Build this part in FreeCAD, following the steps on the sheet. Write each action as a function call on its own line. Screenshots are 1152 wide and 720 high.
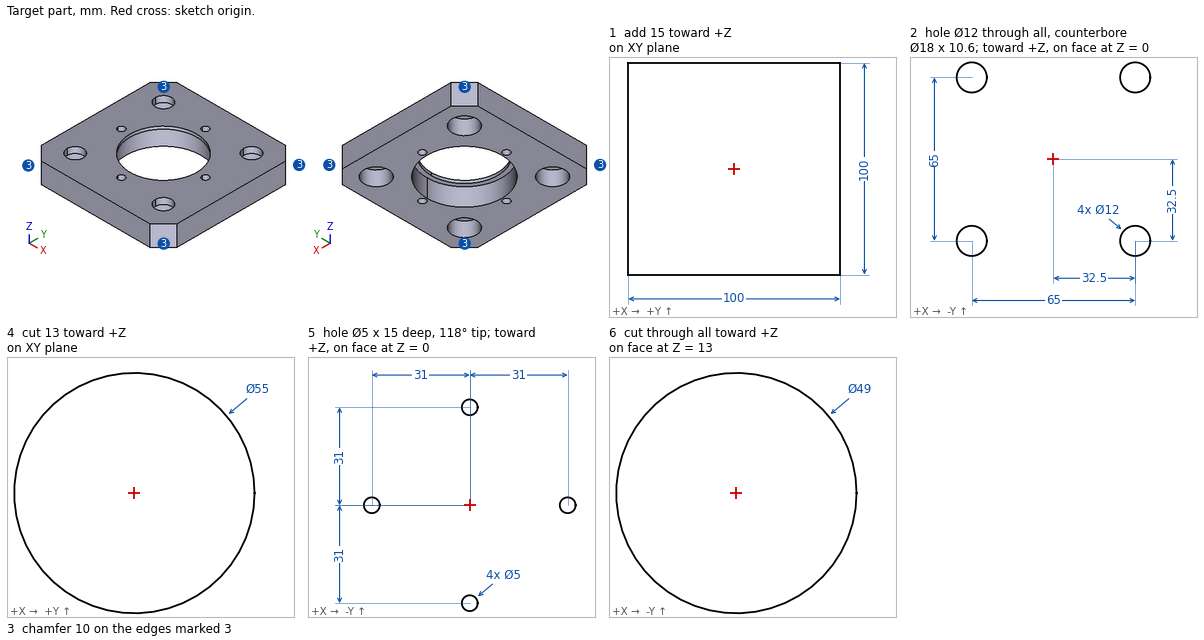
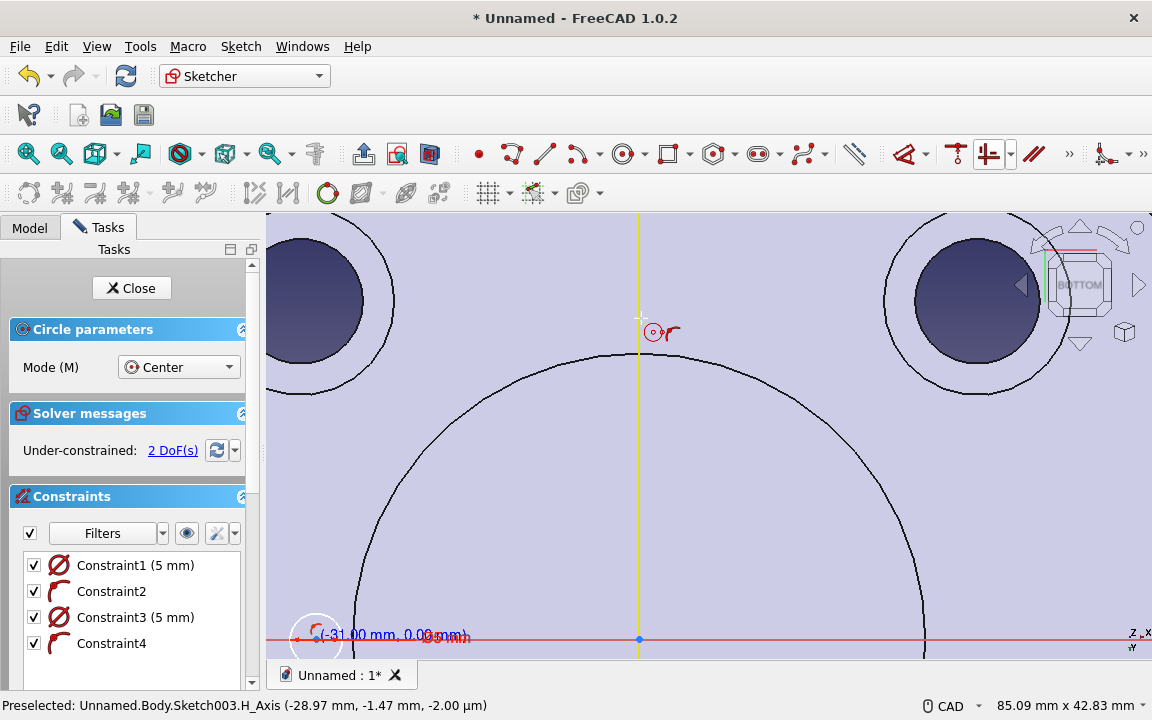
click(639, 317)
move(657, 299)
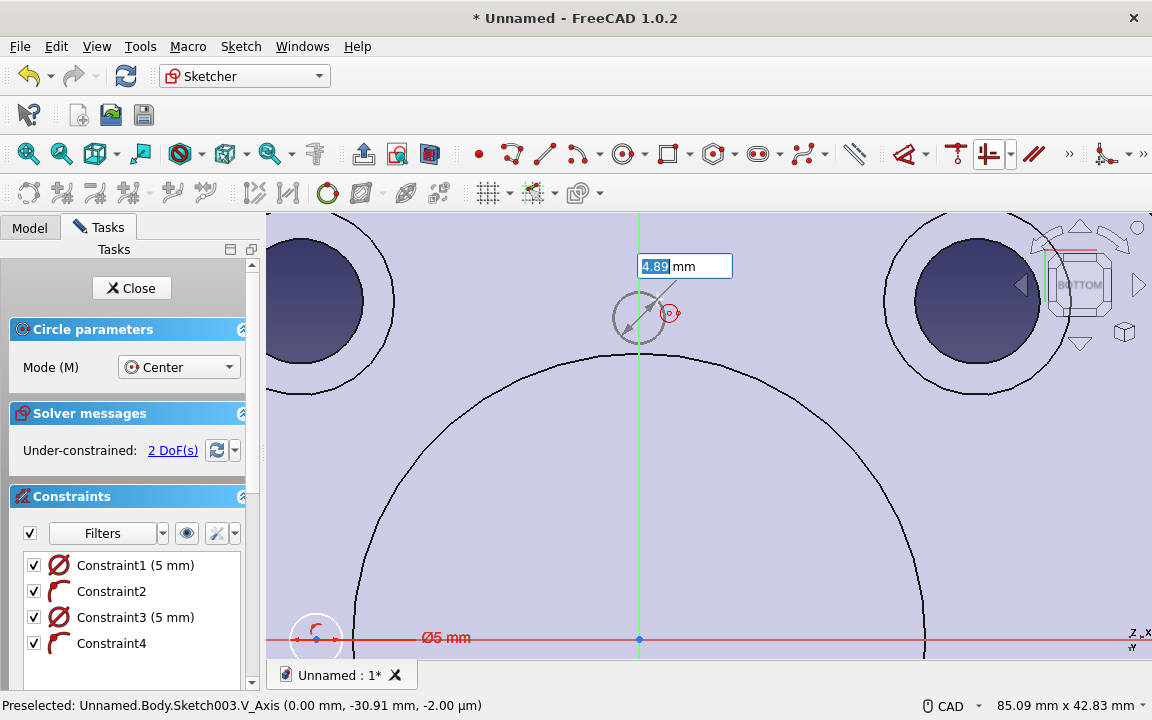
text(5)
key(Return)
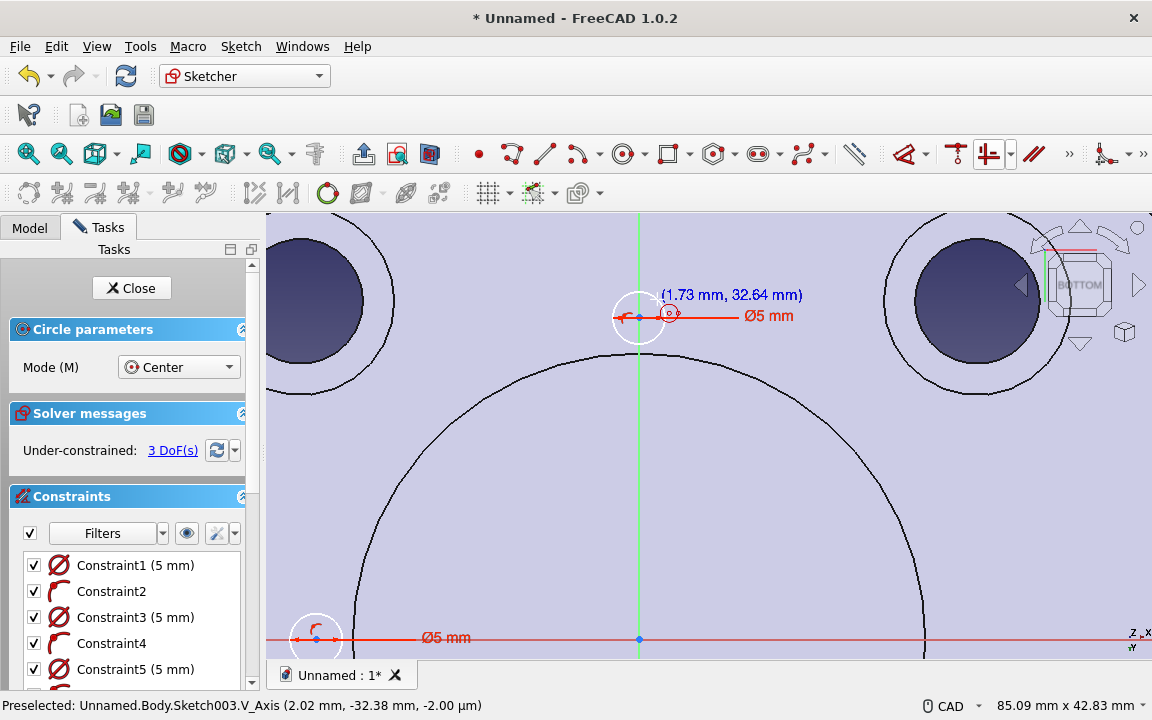
scroll(641, 317, down, 5)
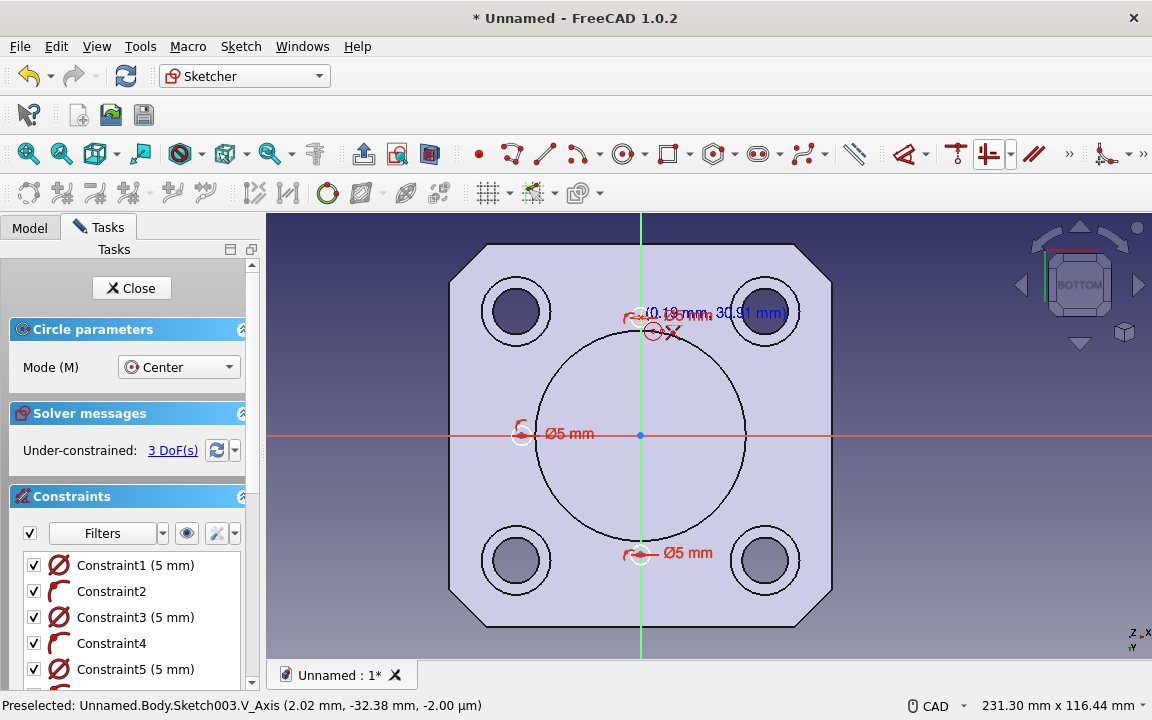
scroll(759, 436, up, 5)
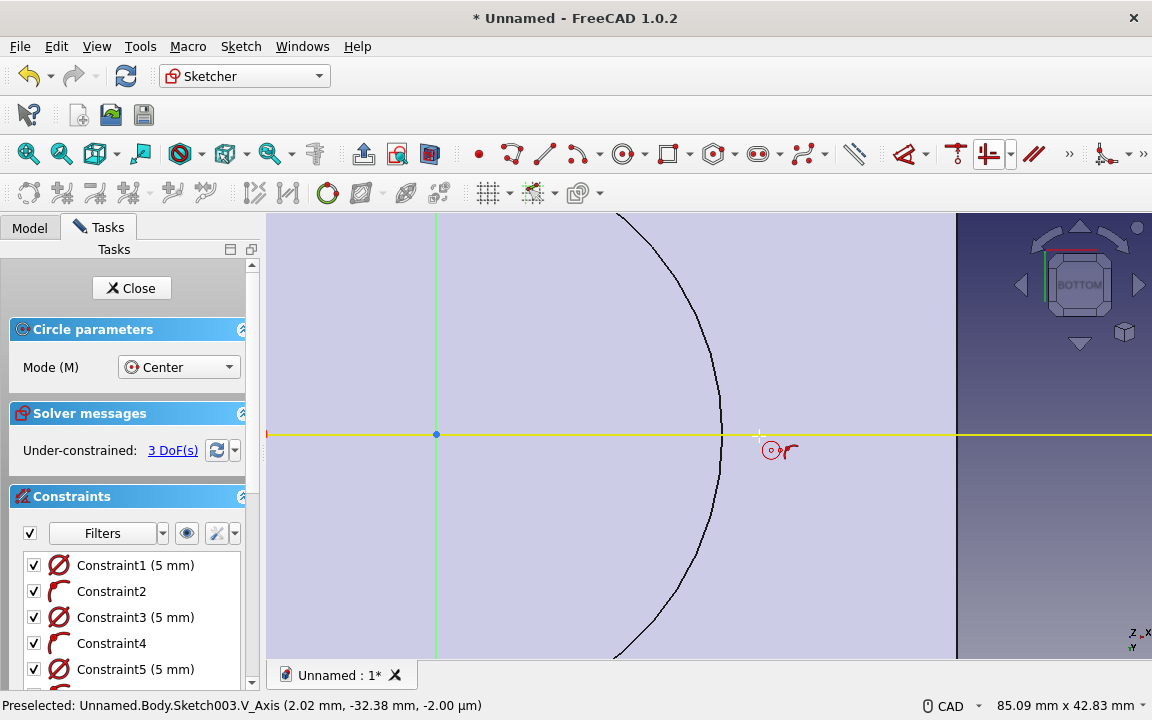
click(759, 435)
move(777, 416)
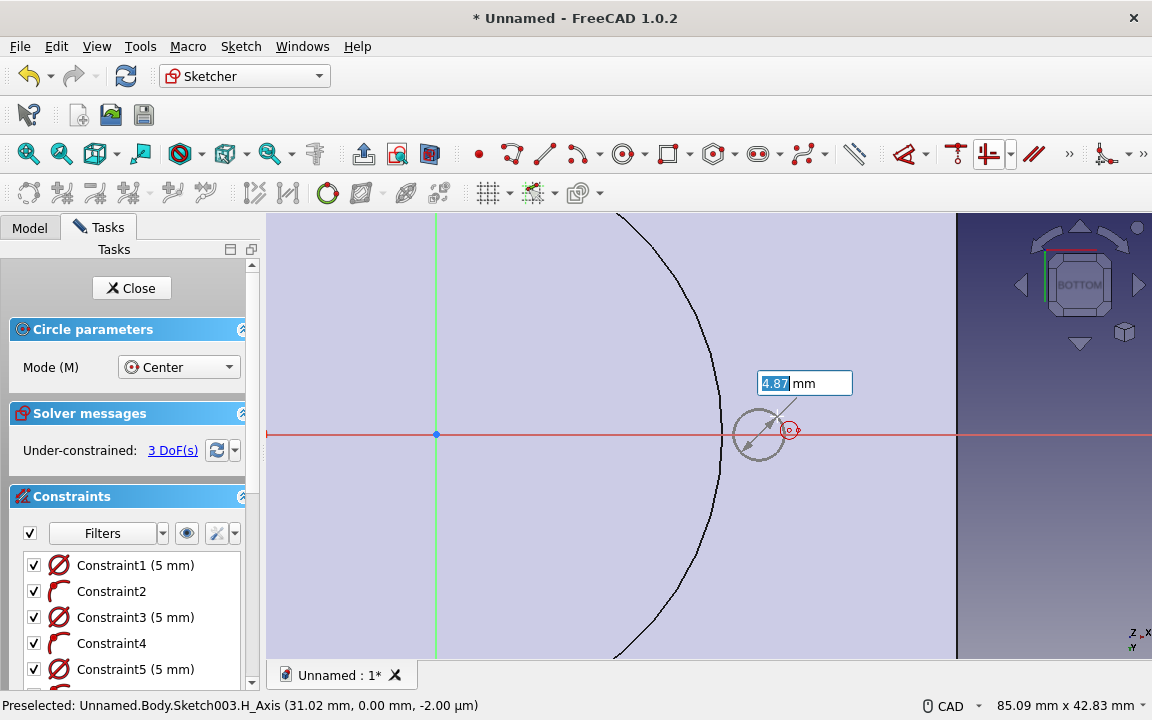
text(5)
key(Return)
key(Escape)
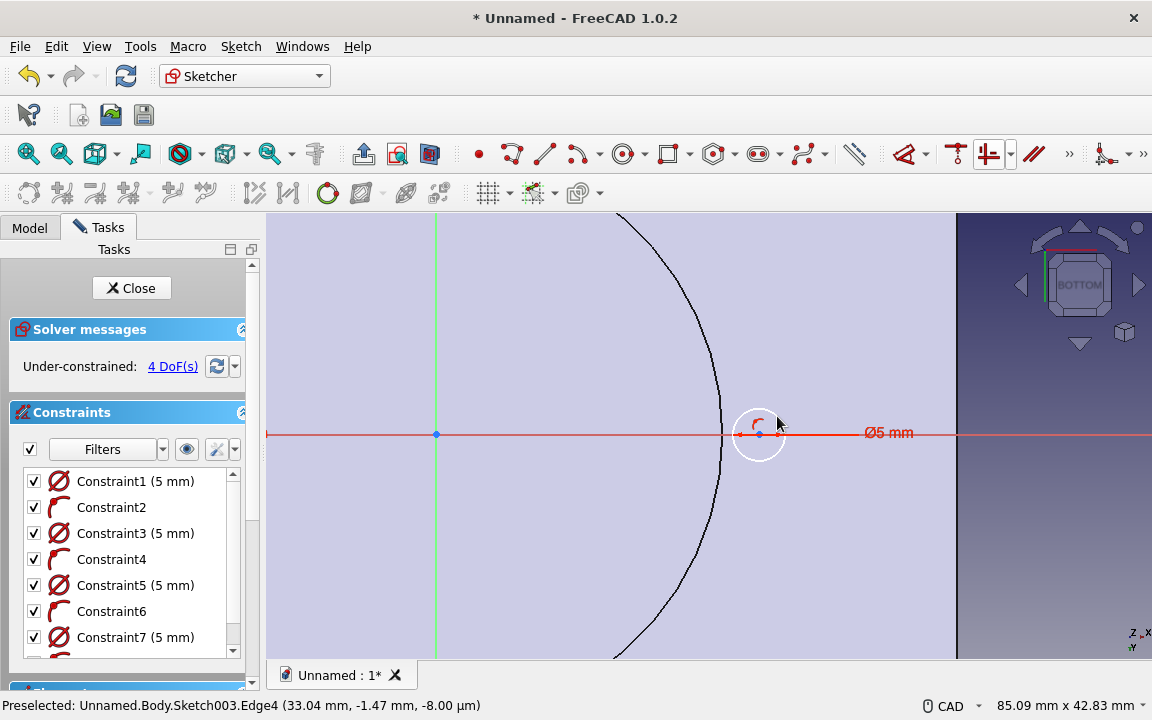
click(904, 154)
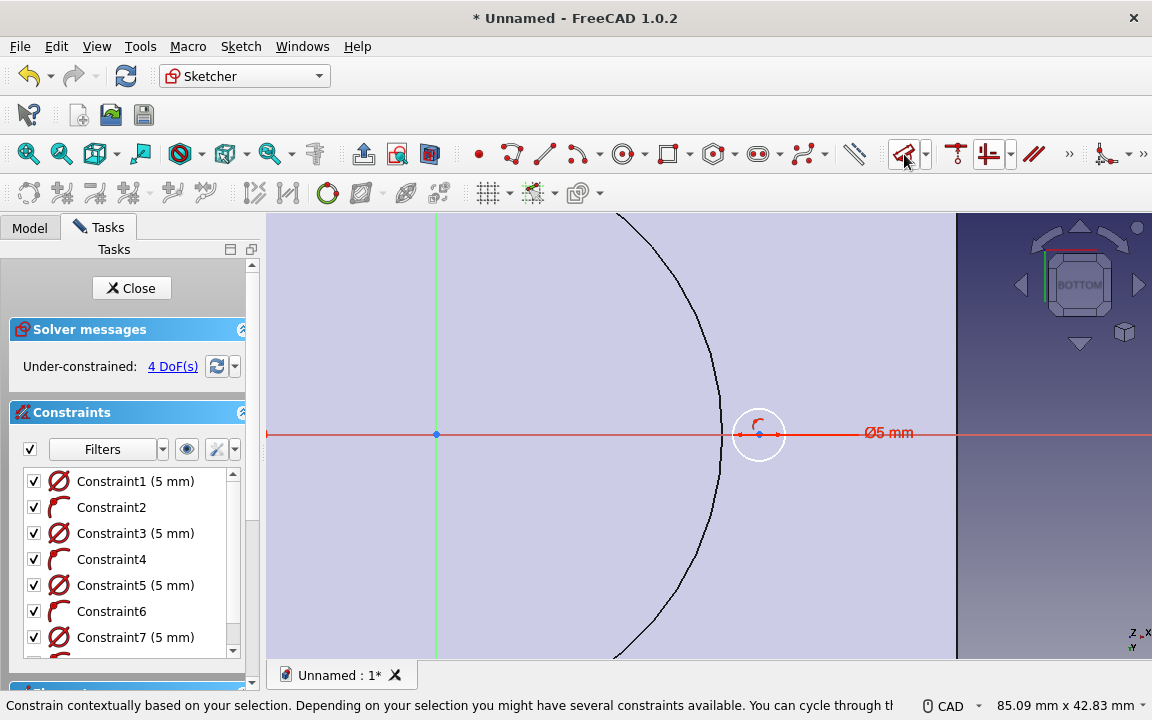
scroll(759, 437, down, 5)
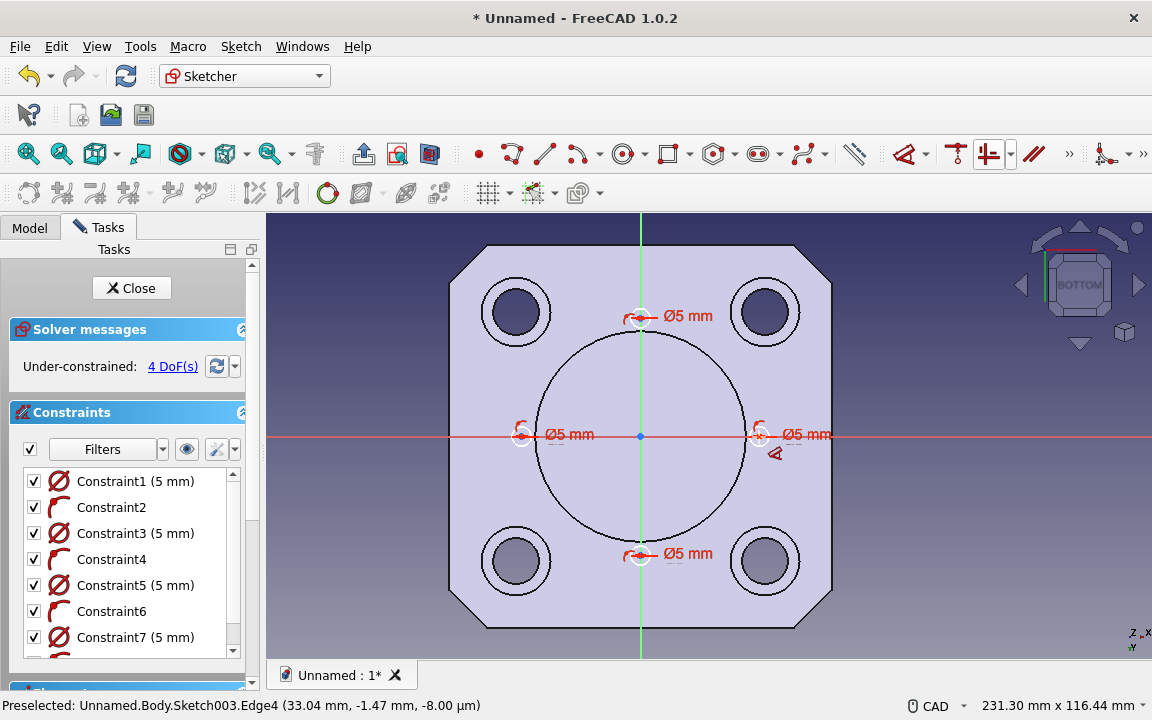
click(641, 556)
click(675, 496)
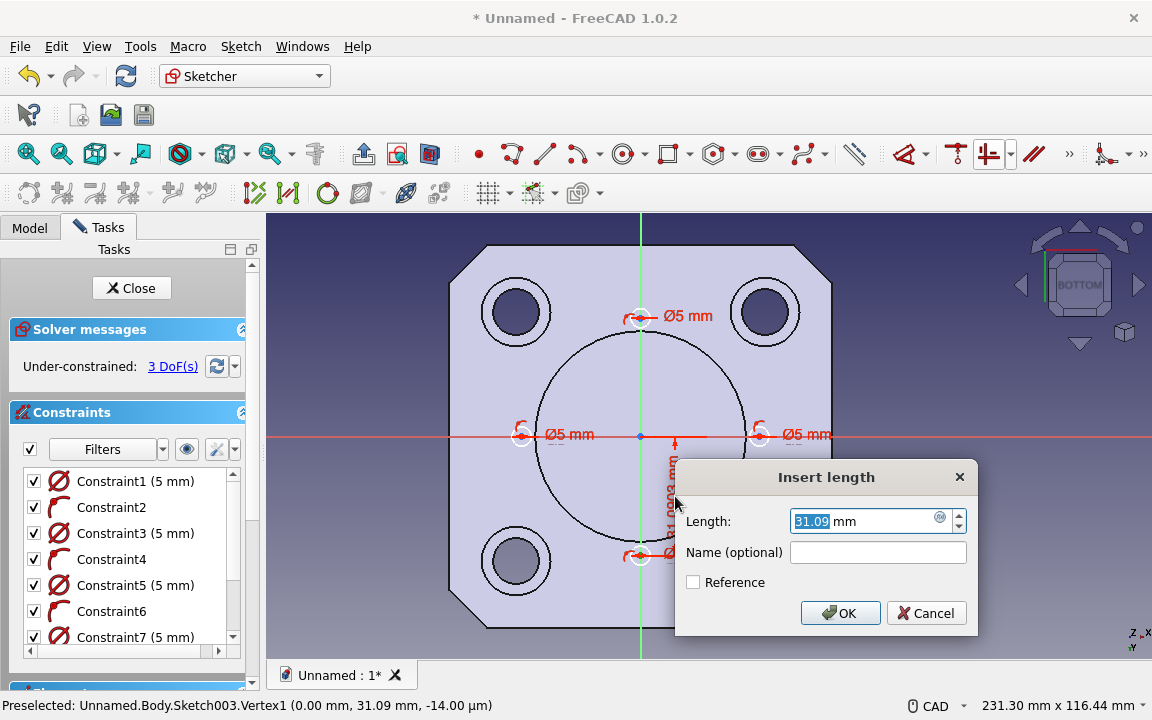
text(31)
key(Return)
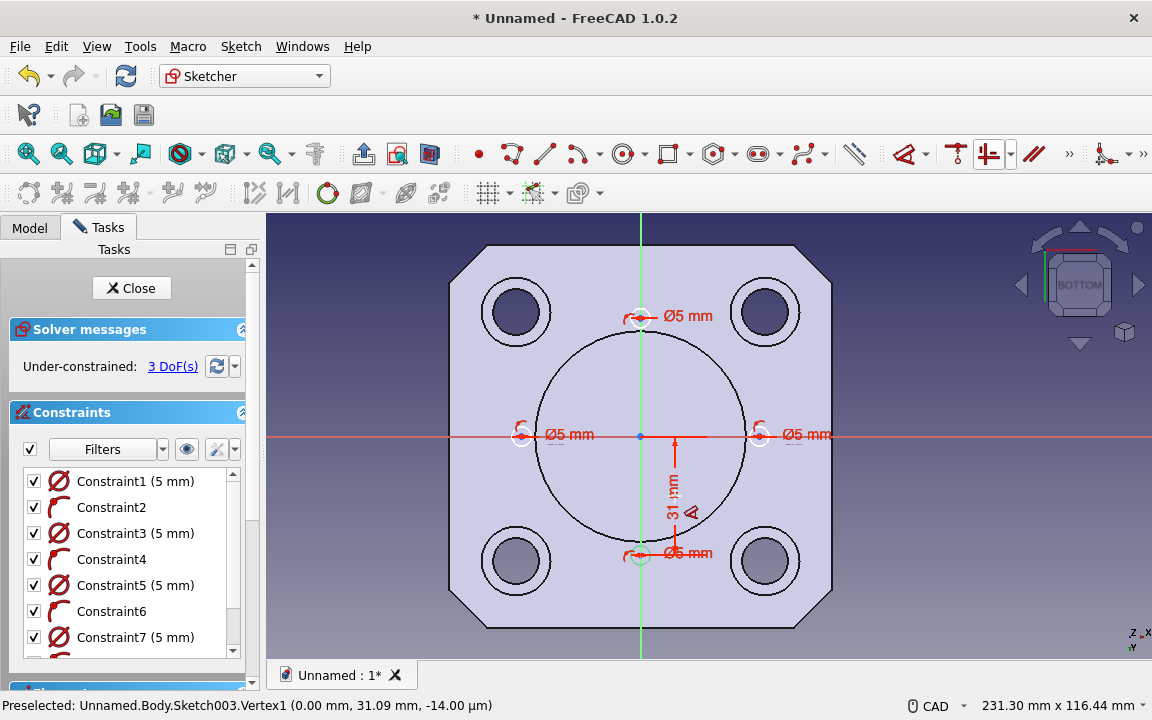
click(522, 437)
click(581, 471)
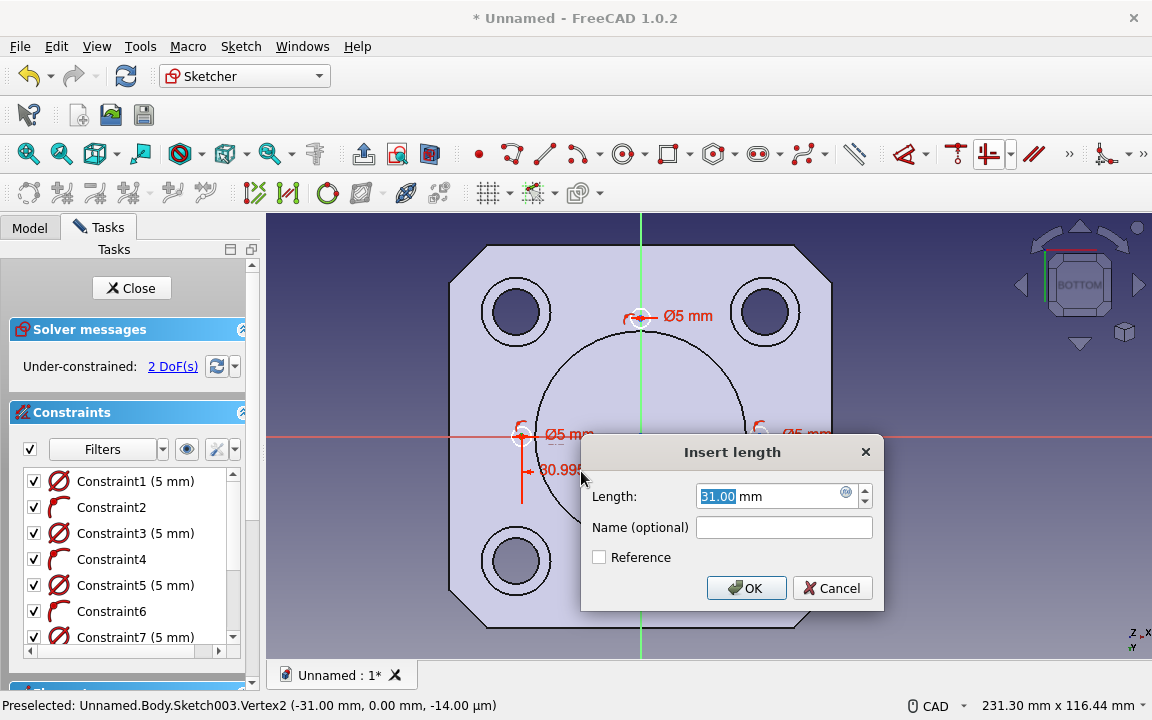
text(31)
key(Return)